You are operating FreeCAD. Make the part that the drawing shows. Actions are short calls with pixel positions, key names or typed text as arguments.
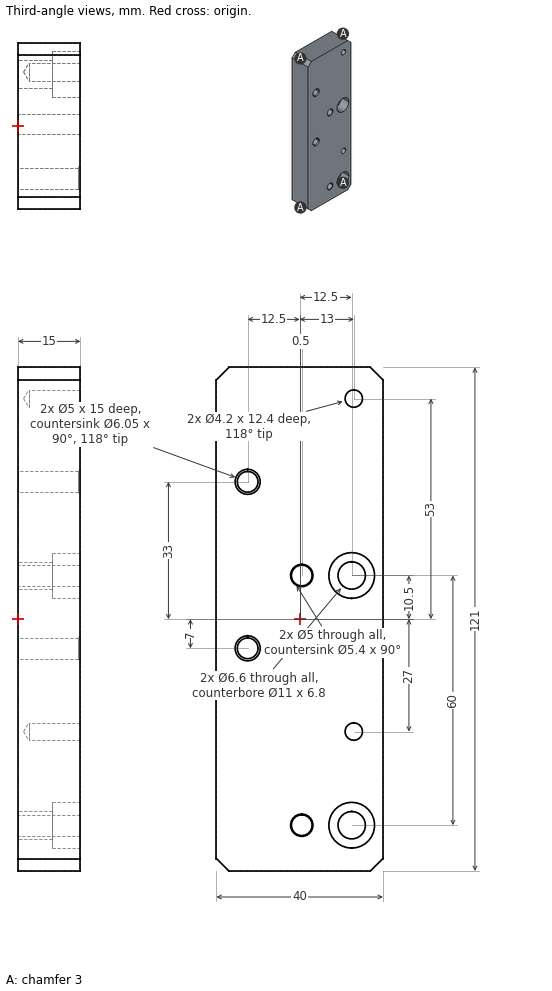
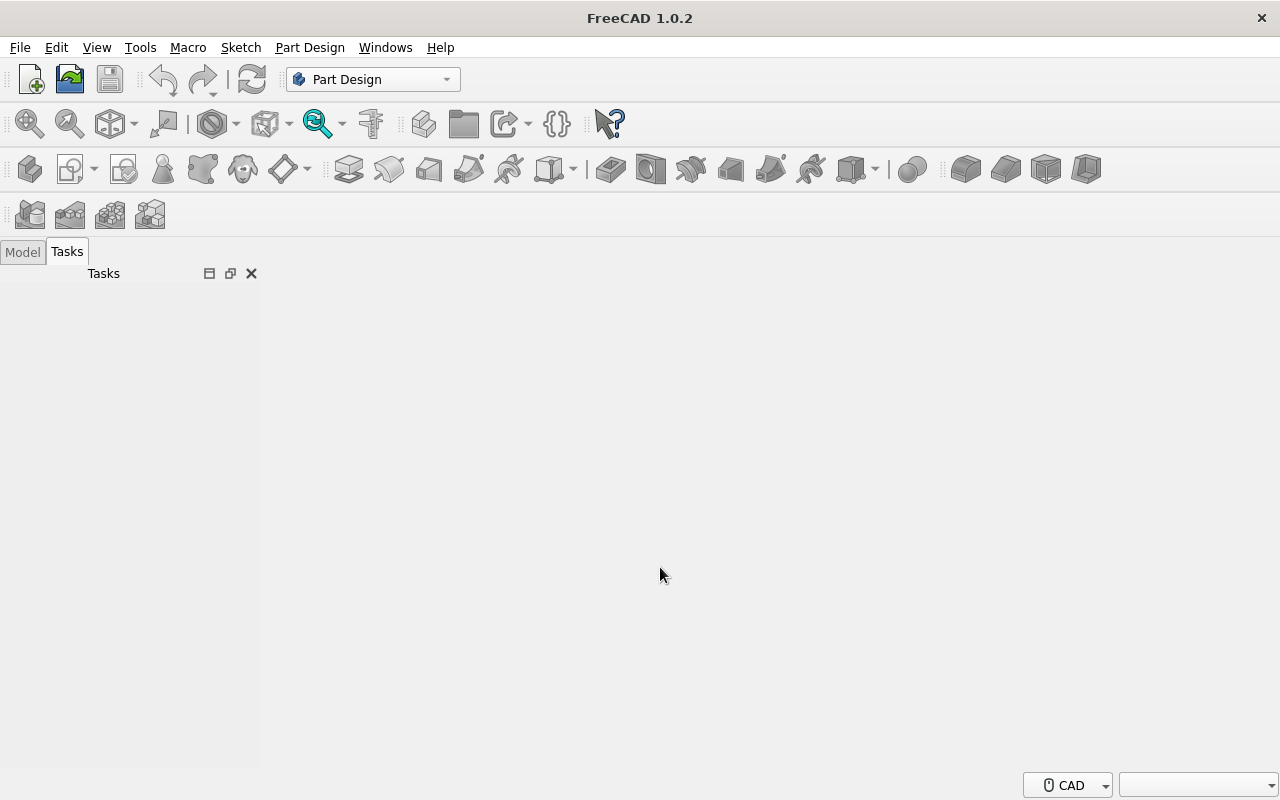
click(30, 80)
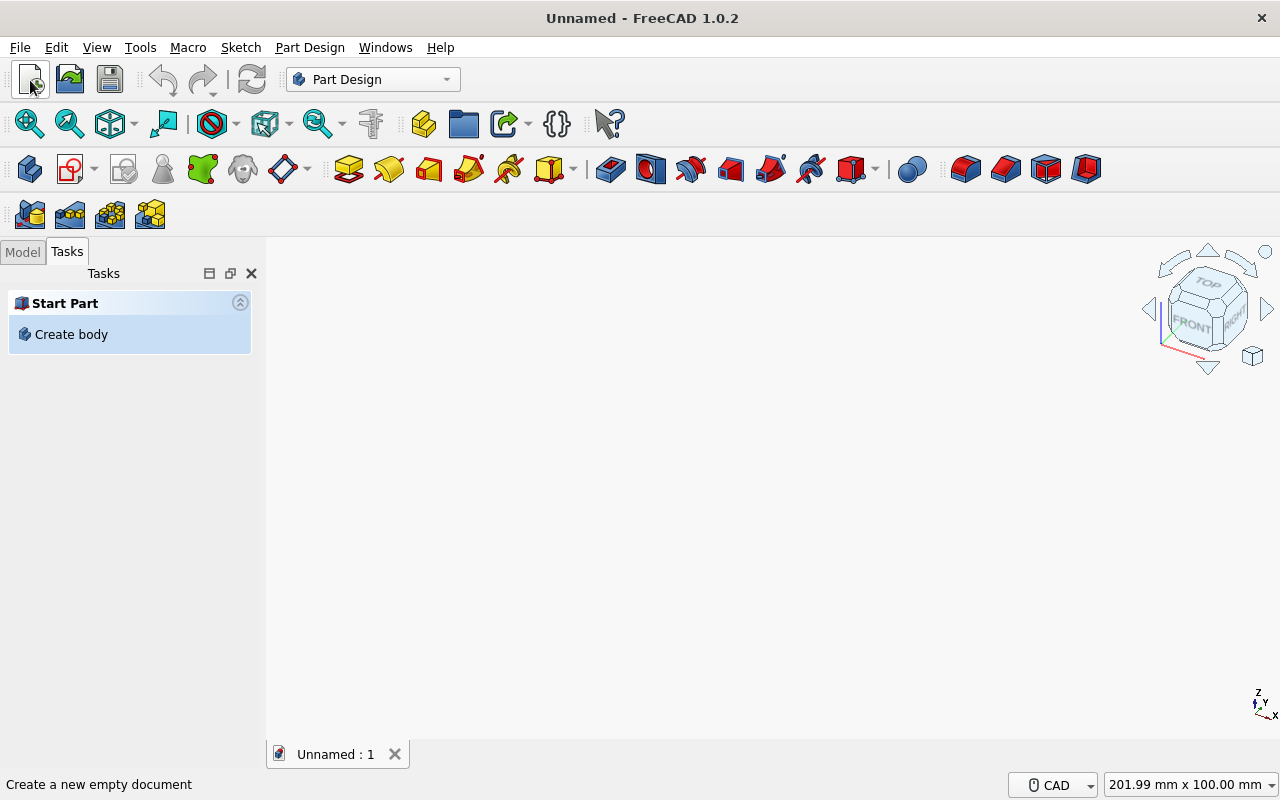
click(70, 170)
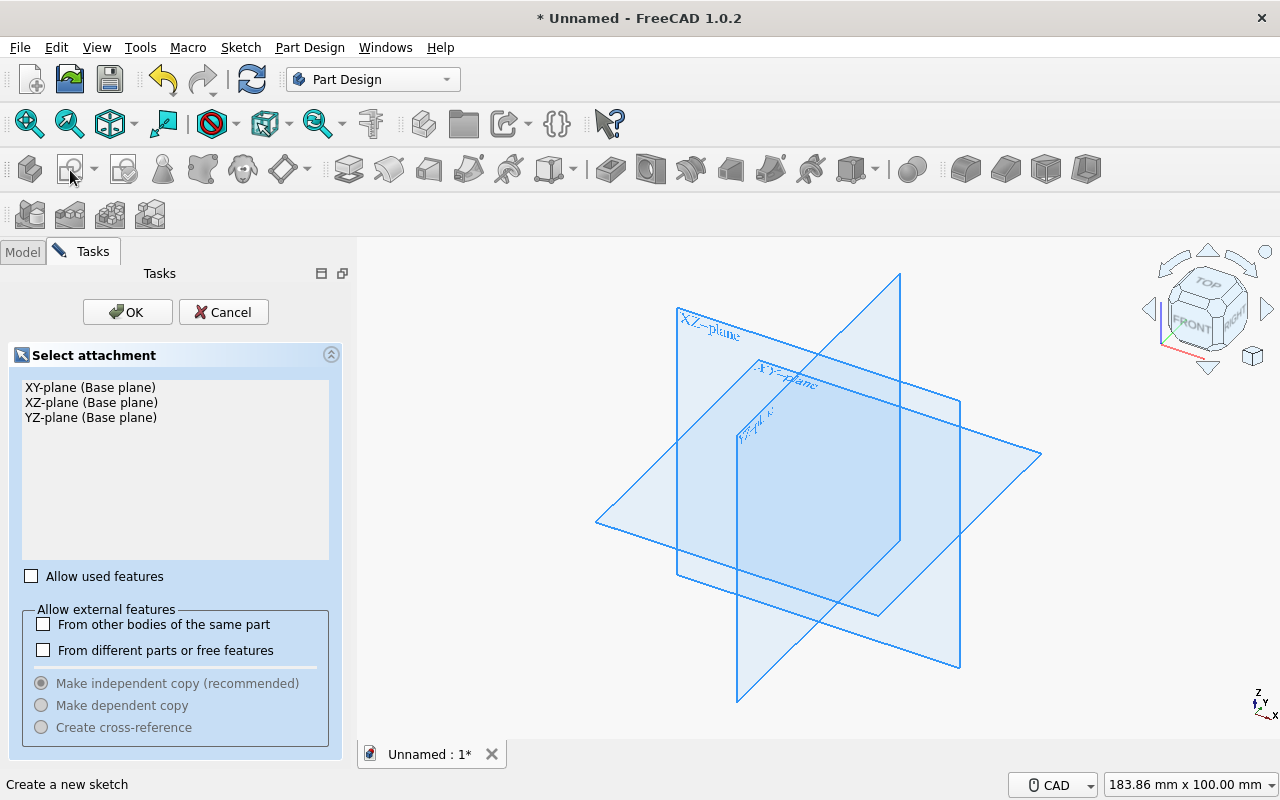
click(82, 418)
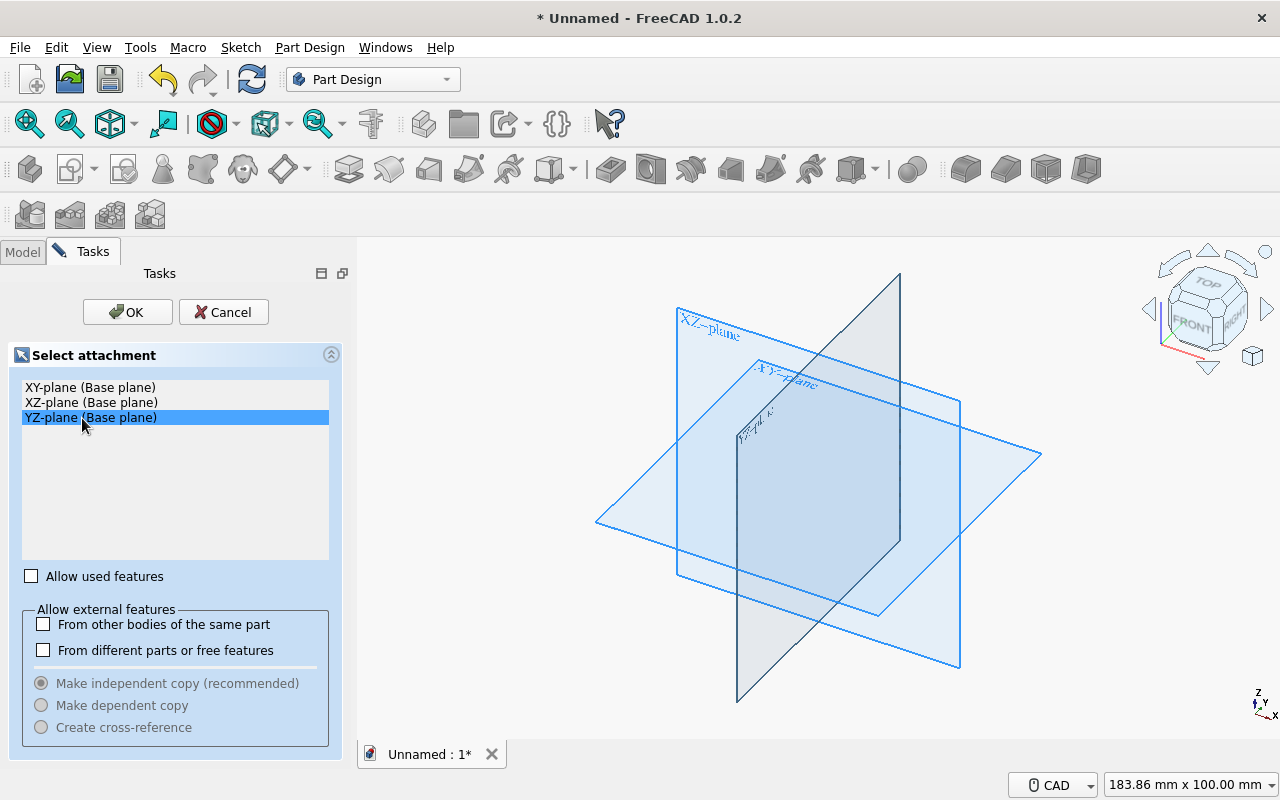
click(128, 312)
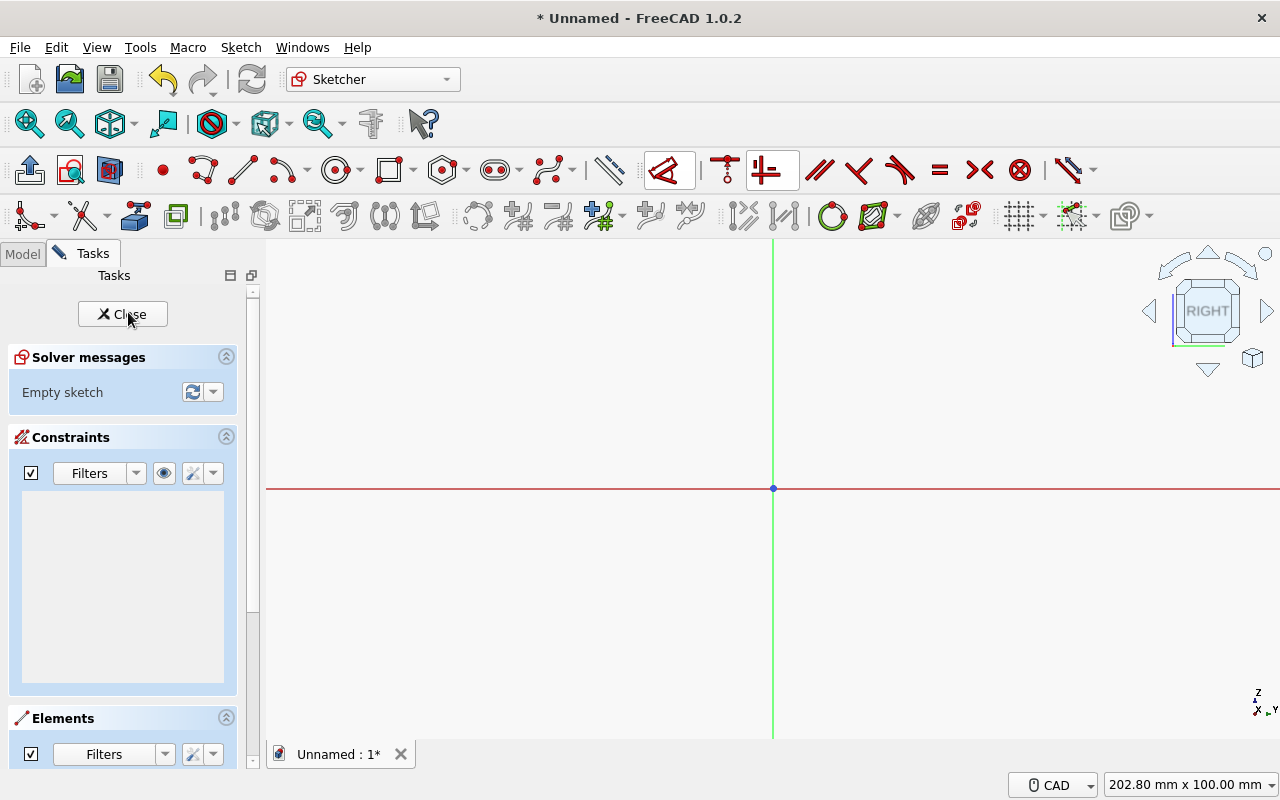
scroll(621, 489, down, 3)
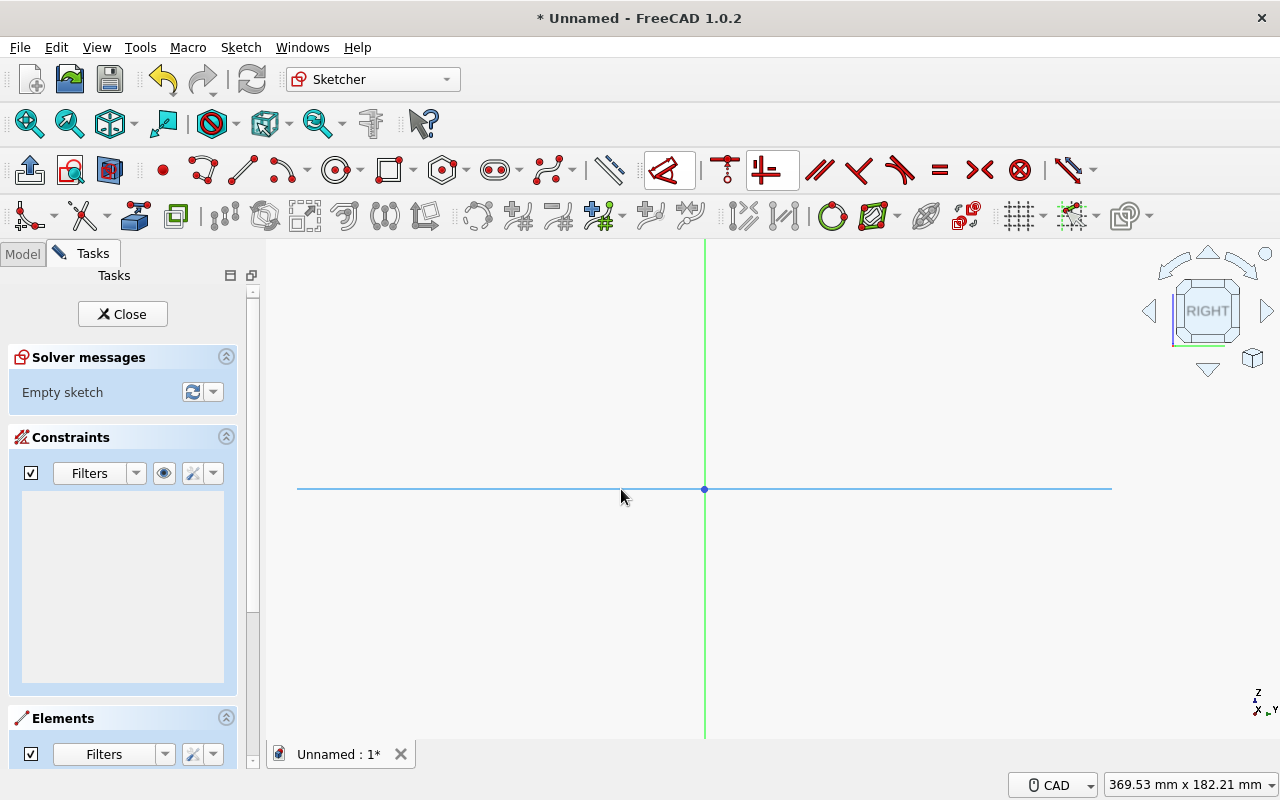
click(416, 170)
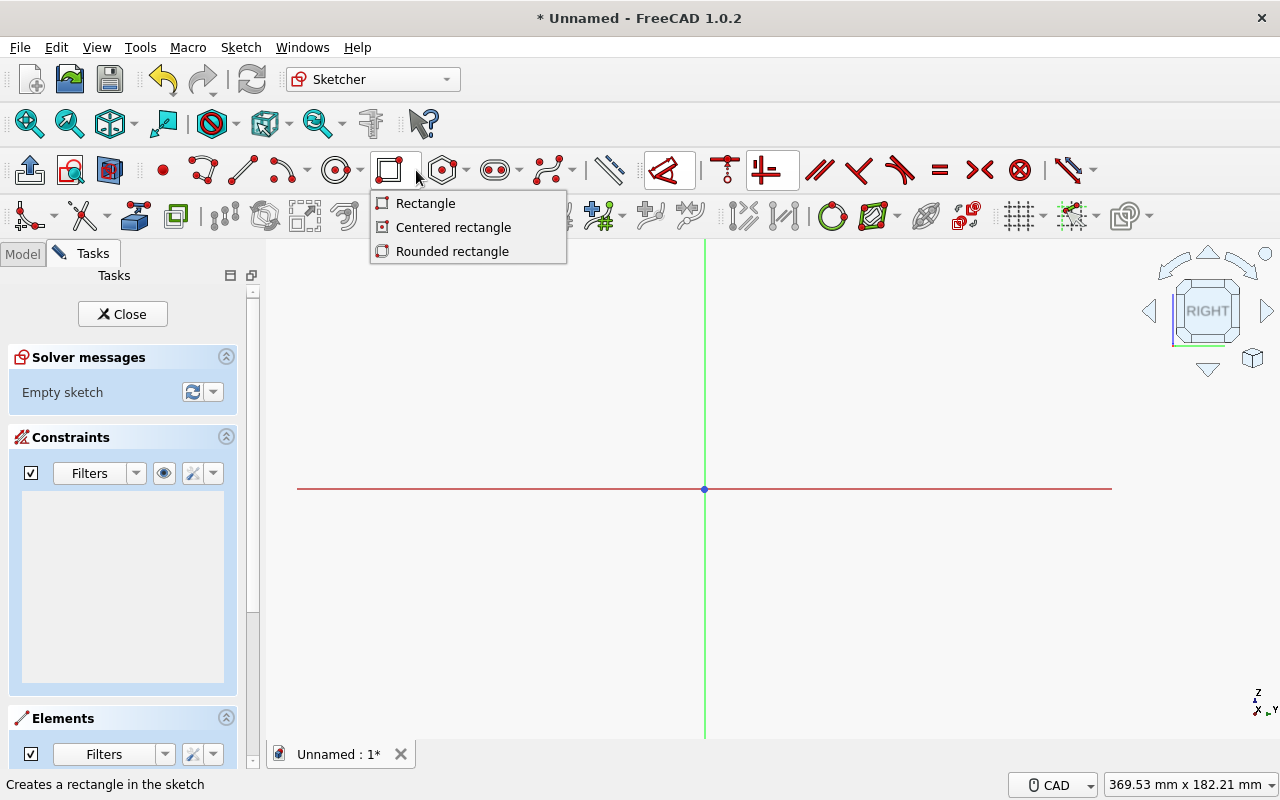
click(468, 227)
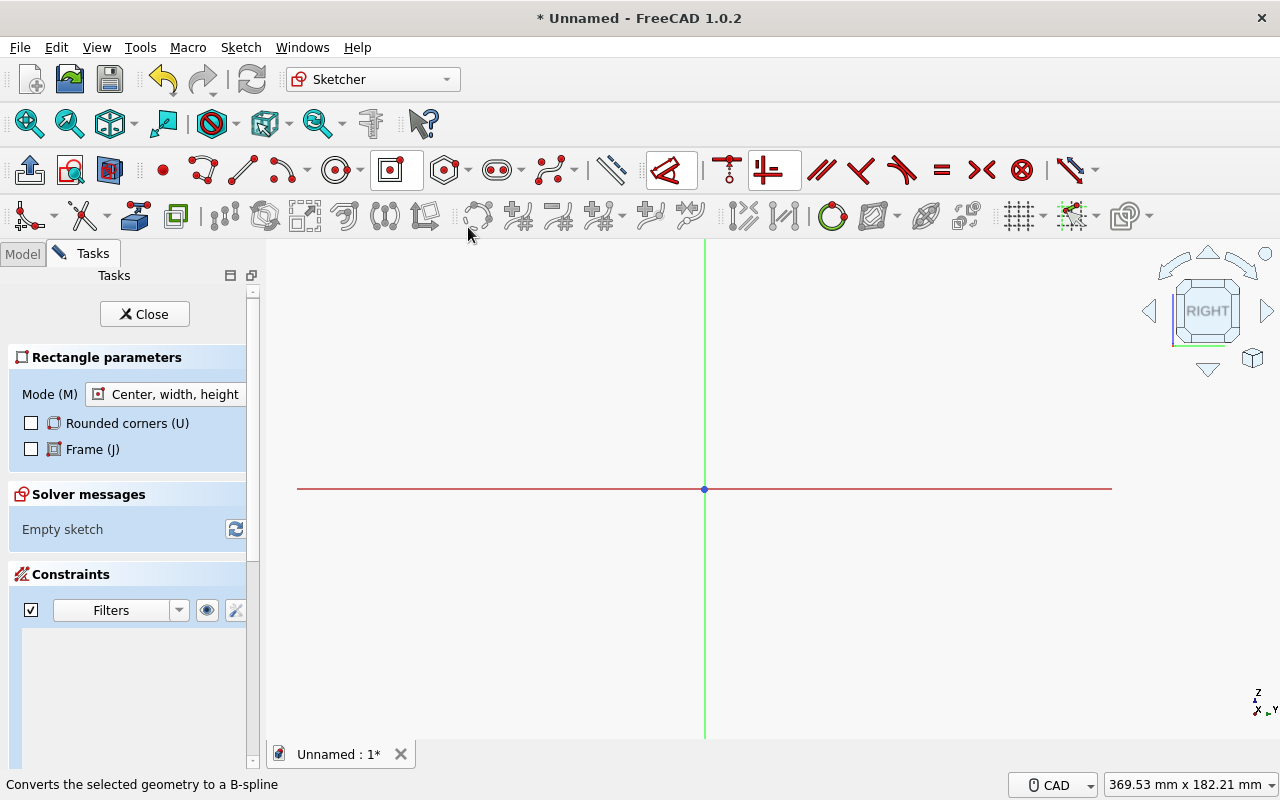
click(705, 489)
move(759, 323)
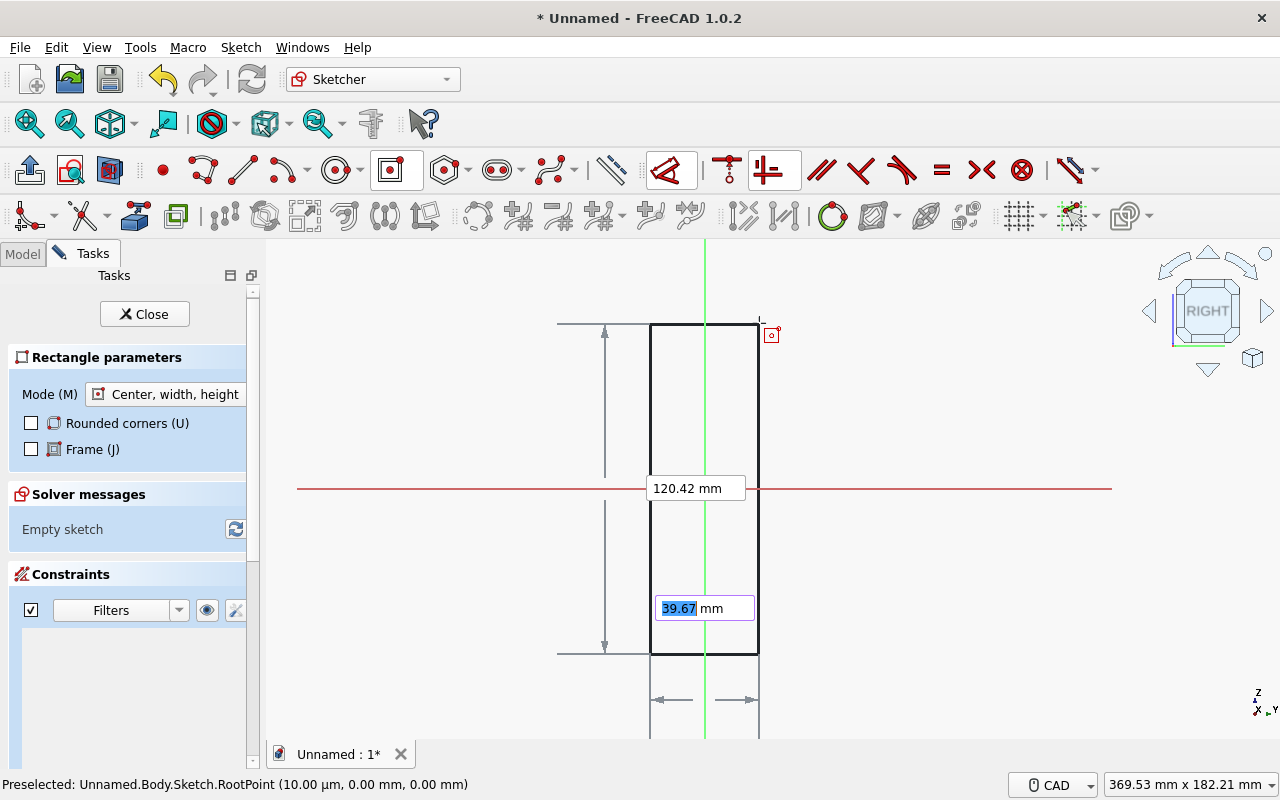
text(40)
key(Tab)
text(121)
key(Return)
key(Escape)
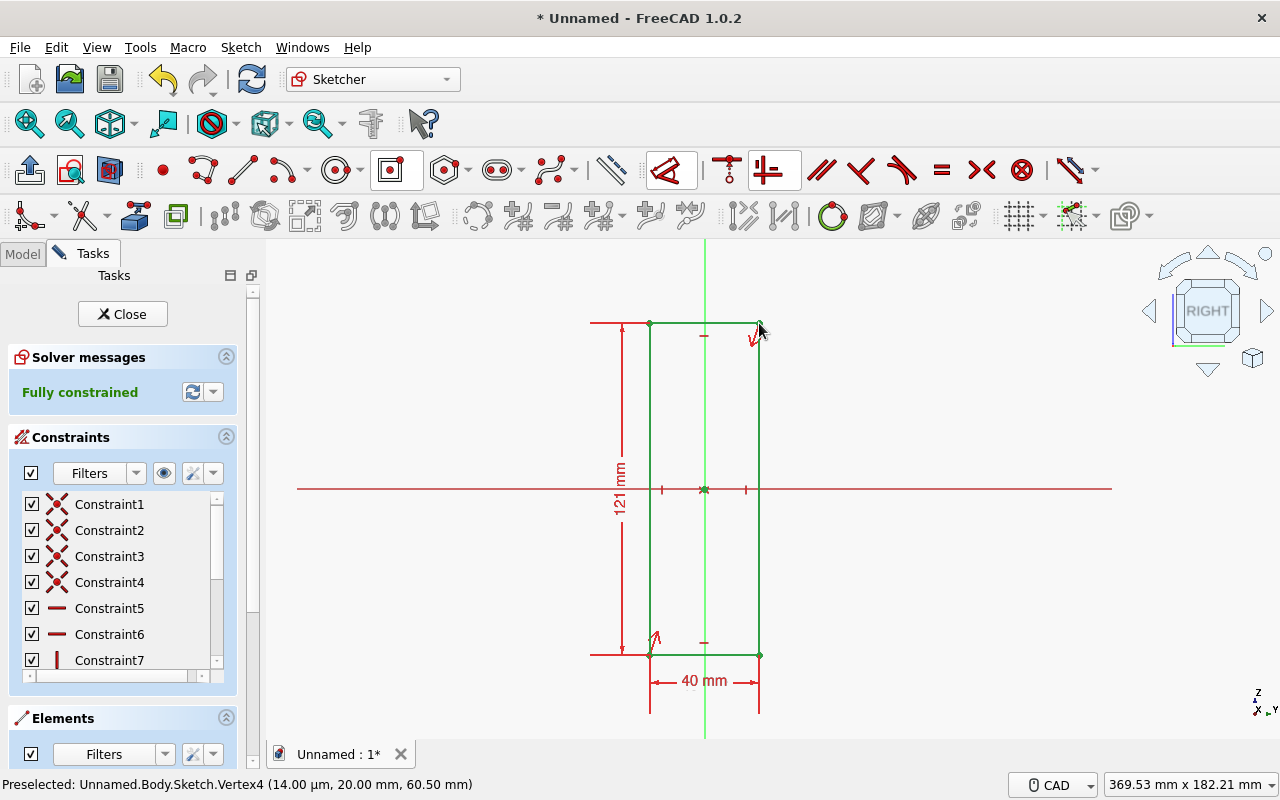
click(123, 314)